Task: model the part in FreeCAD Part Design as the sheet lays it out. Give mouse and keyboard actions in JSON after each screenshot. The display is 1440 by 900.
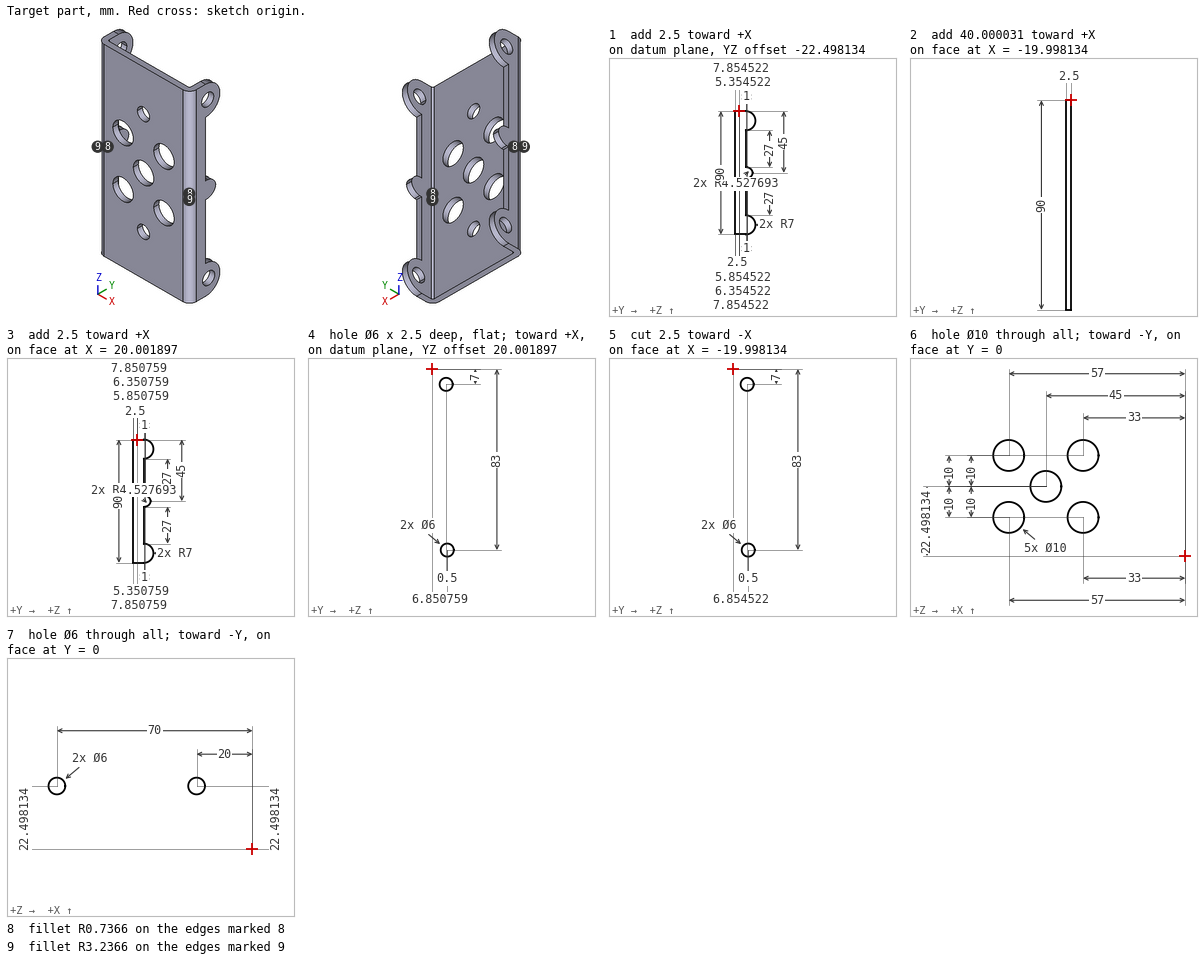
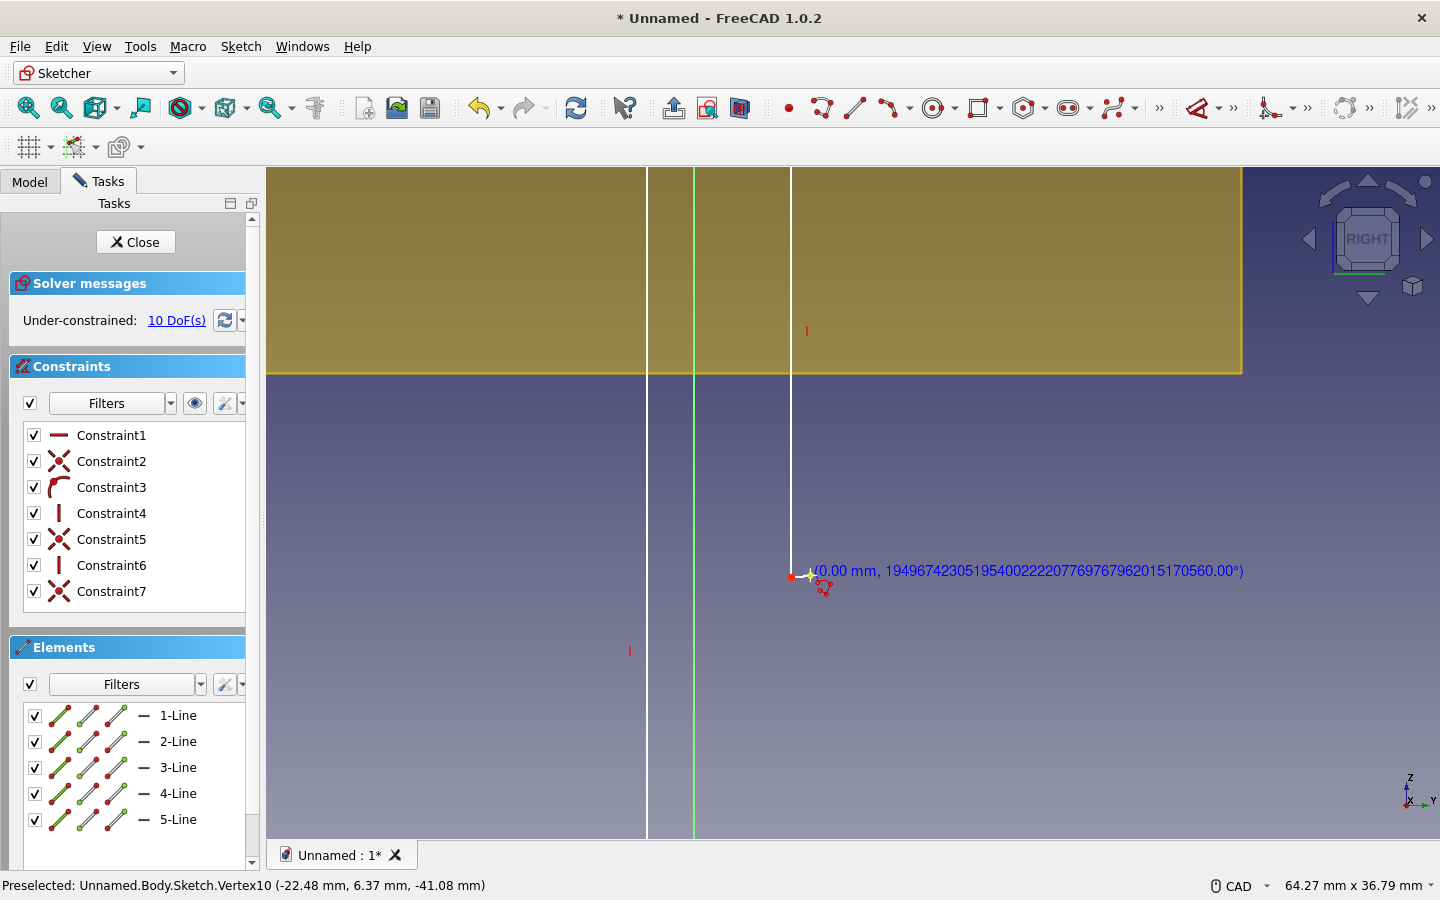
{"action": "scroll", "coordinate": [785, 456], "scroll_direction": "down", "scroll_amount": 7}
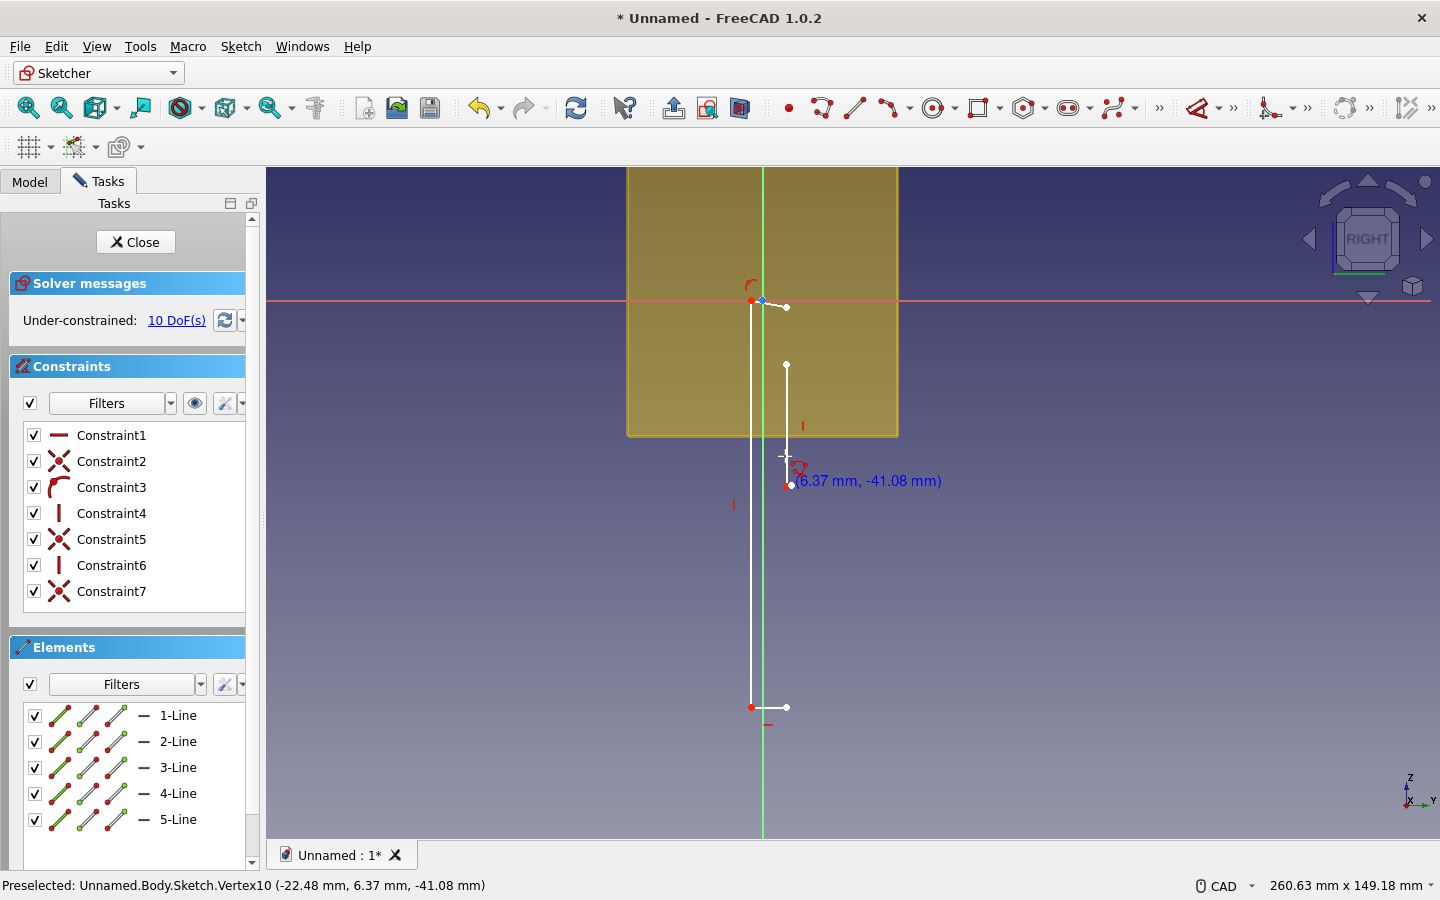
{"action": "left_click", "coordinate": [791, 522]}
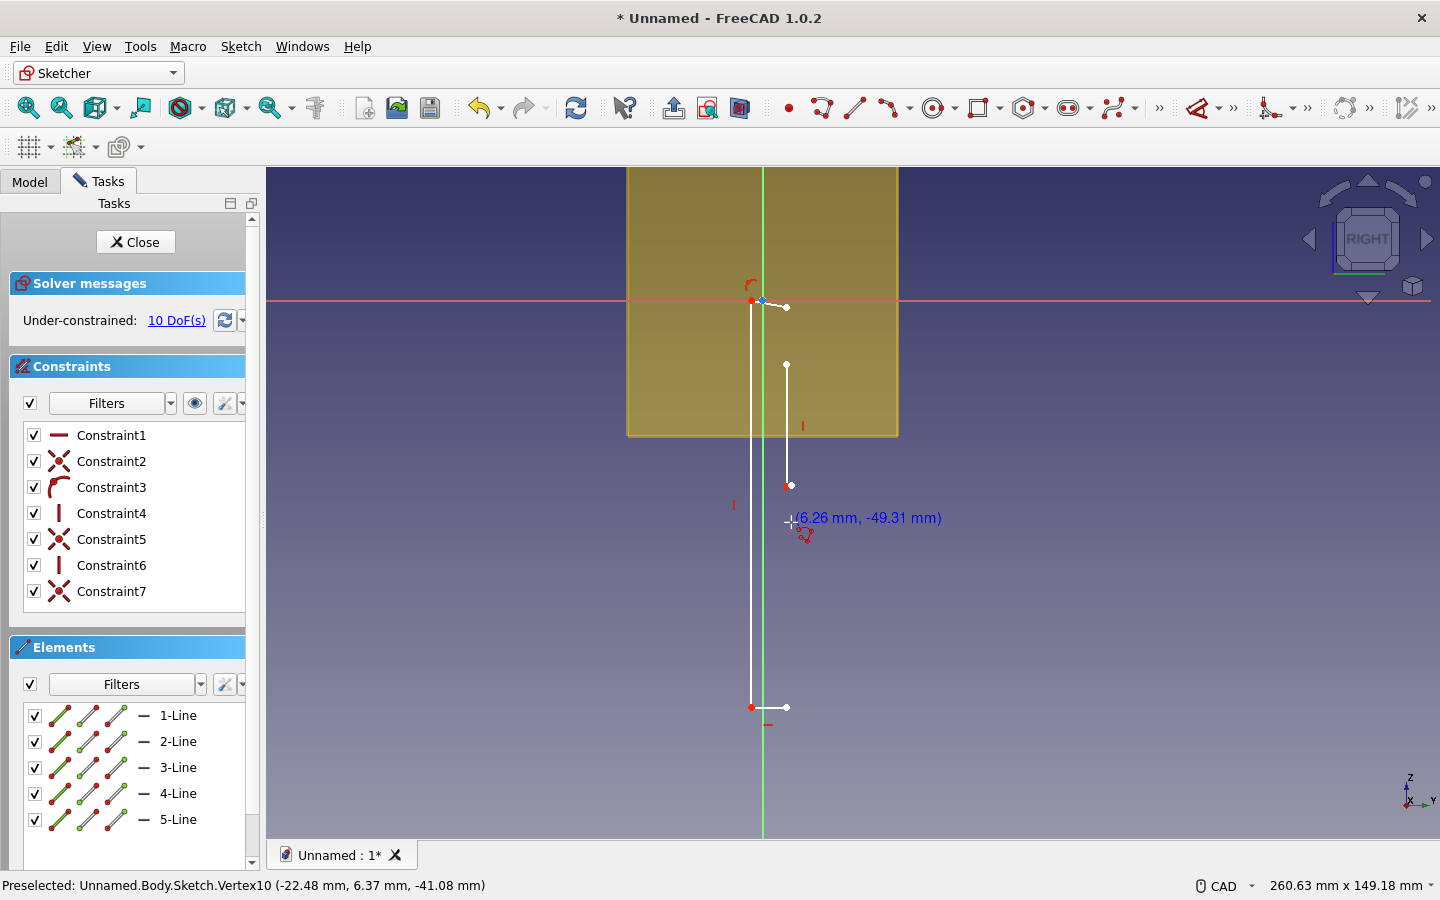
{"action": "scroll", "coordinate": [787, 522], "scroll_direction": "up", "scroll_amount": 7}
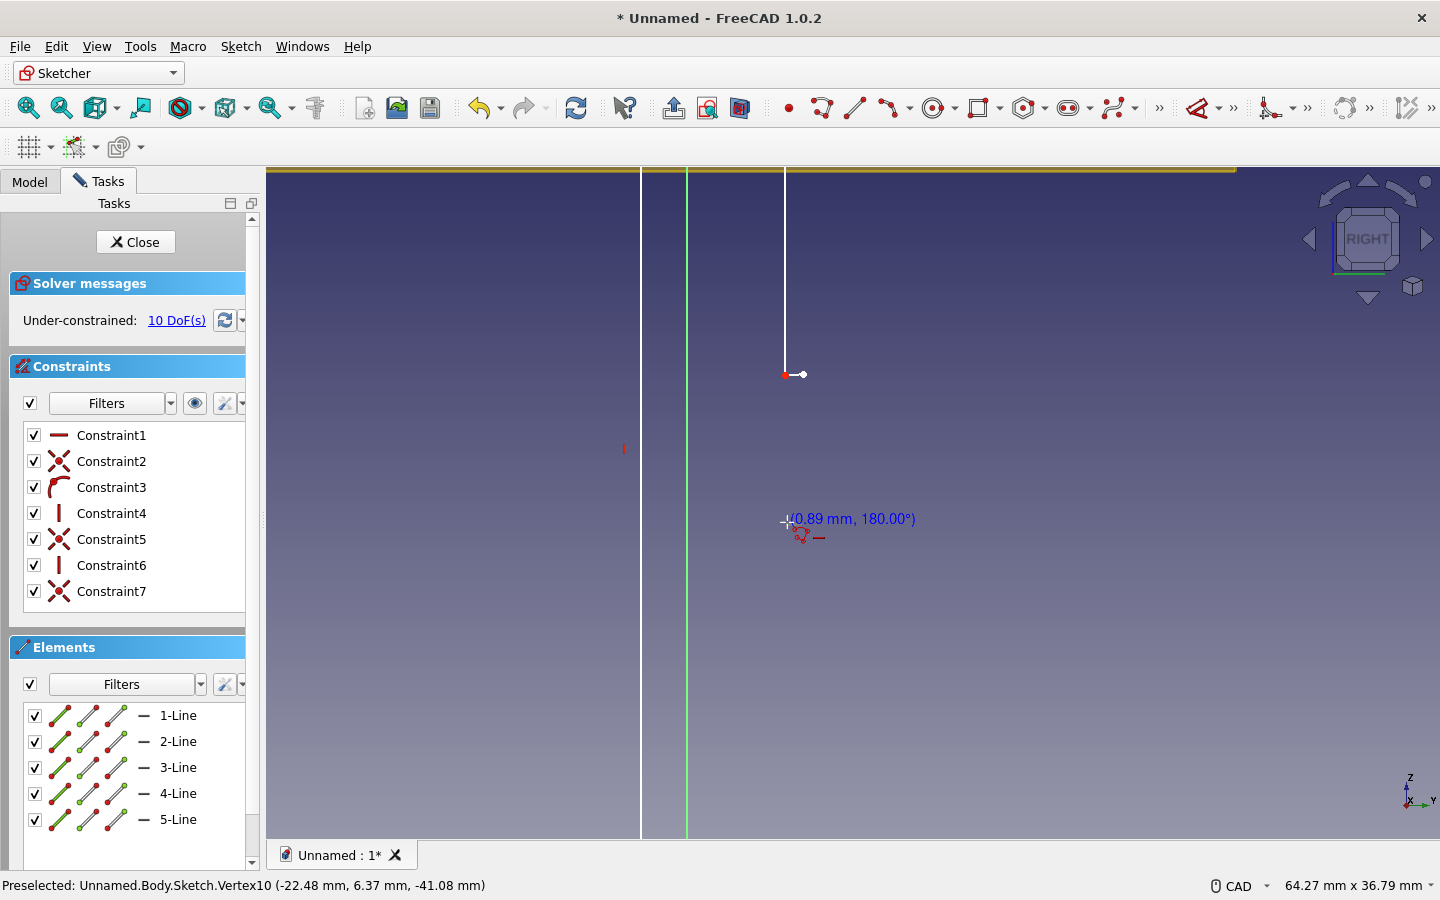
{"action": "left_click", "coordinate": [785, 520]}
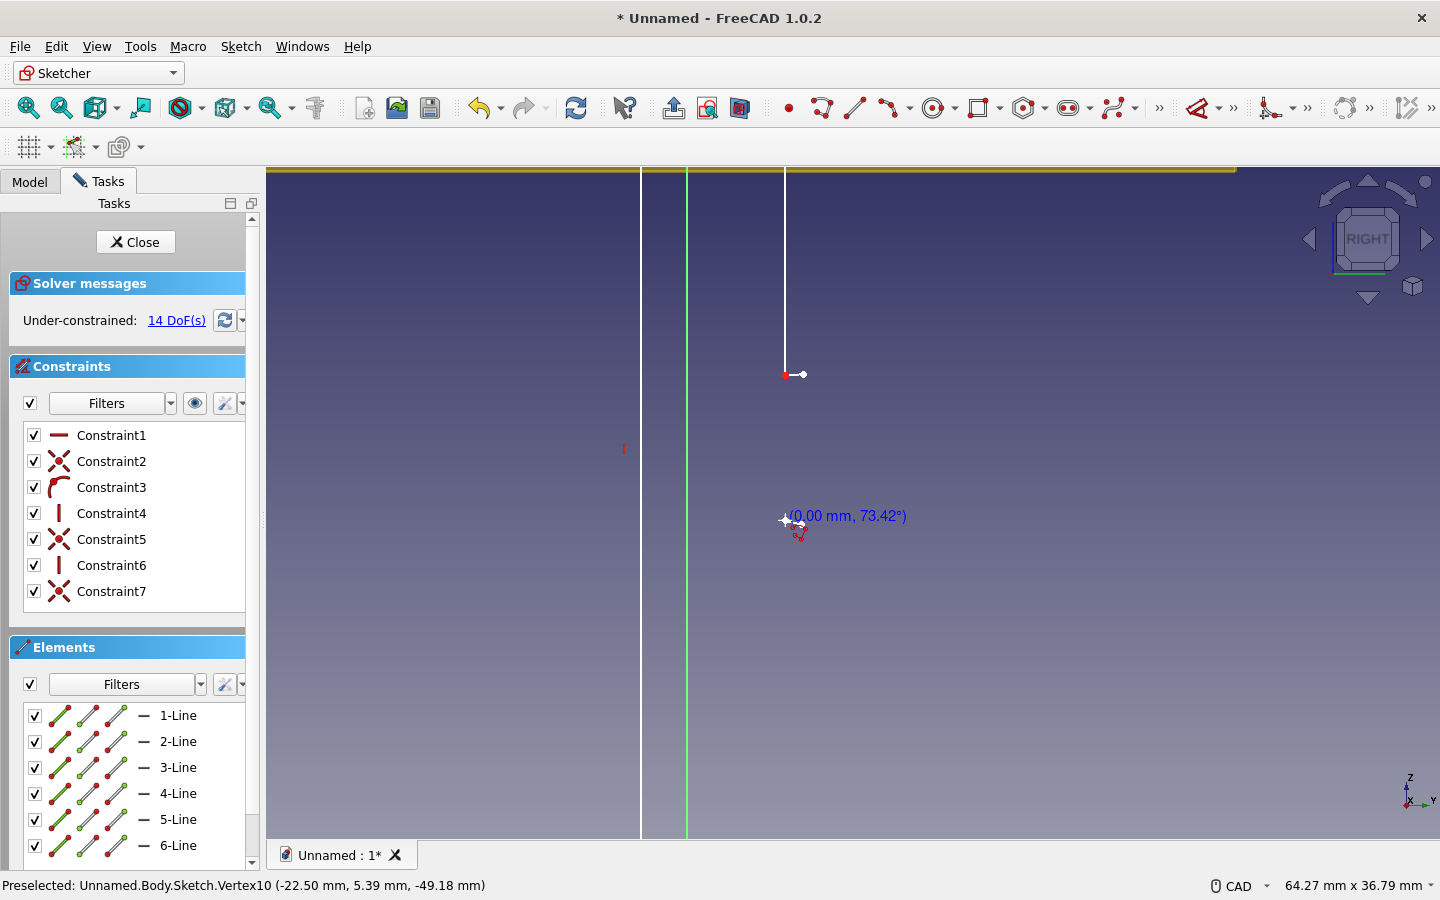
{"action": "scroll", "coordinate": [787, 522], "scroll_direction": "down", "scroll_amount": 7}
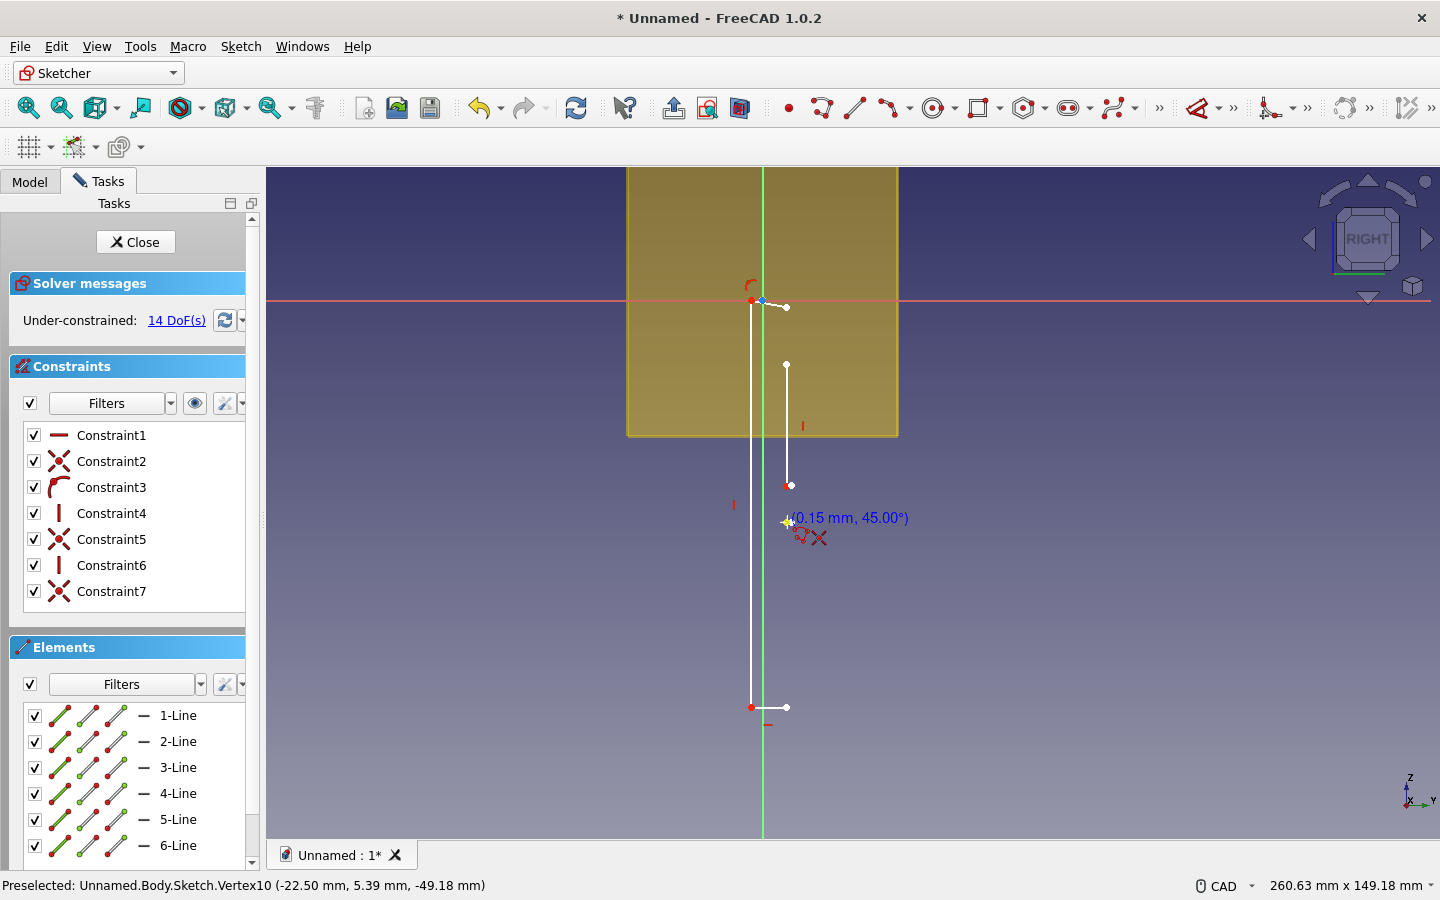
{"action": "left_click", "coordinate": [787, 643]}
{"action": "right_click", "coordinate": [787, 643]}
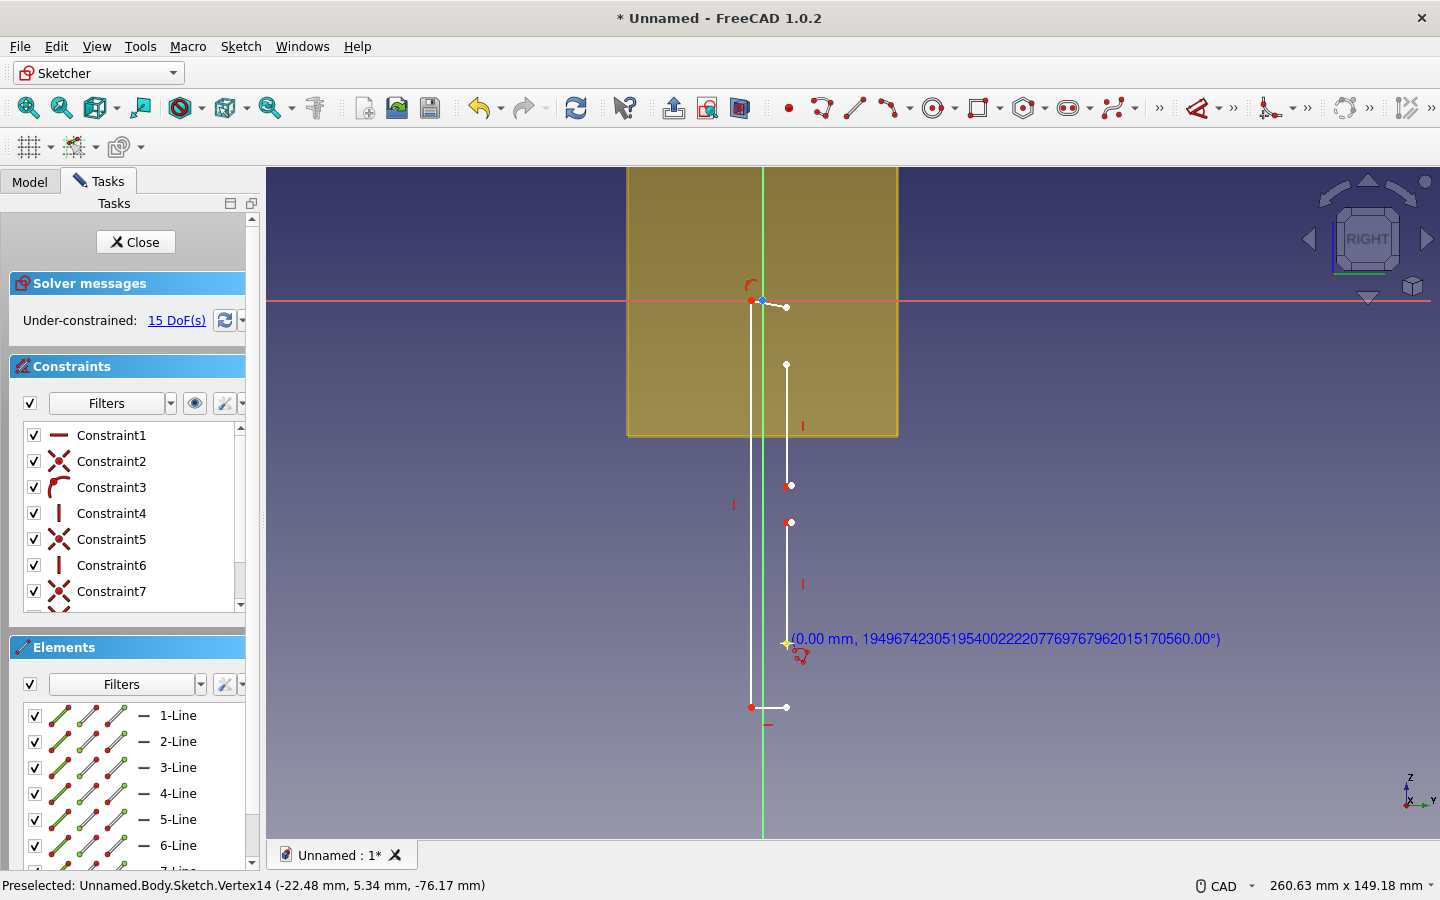
{"action": "left_click", "coordinate": [888, 108]}